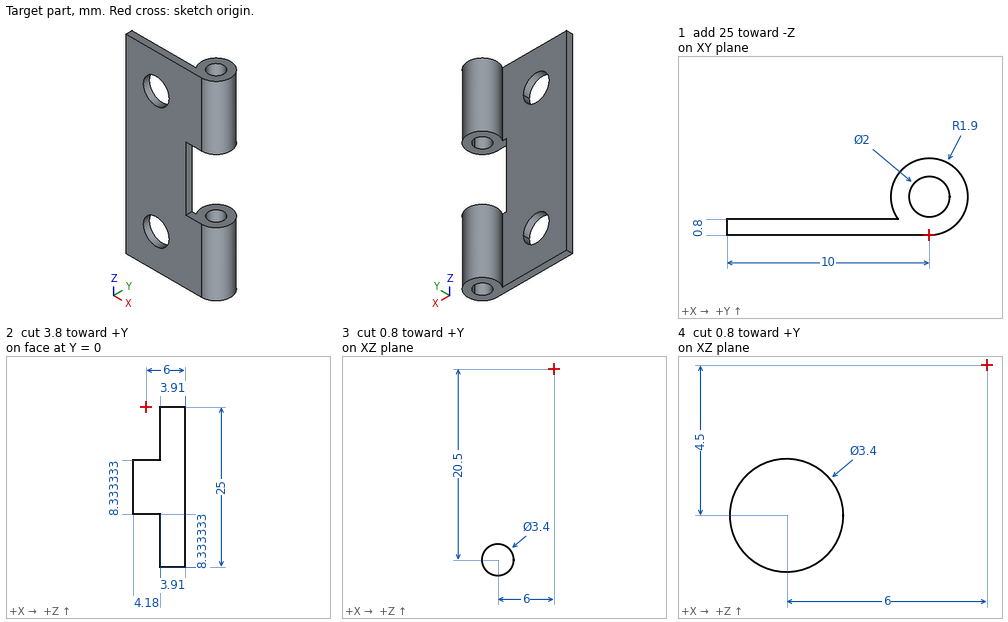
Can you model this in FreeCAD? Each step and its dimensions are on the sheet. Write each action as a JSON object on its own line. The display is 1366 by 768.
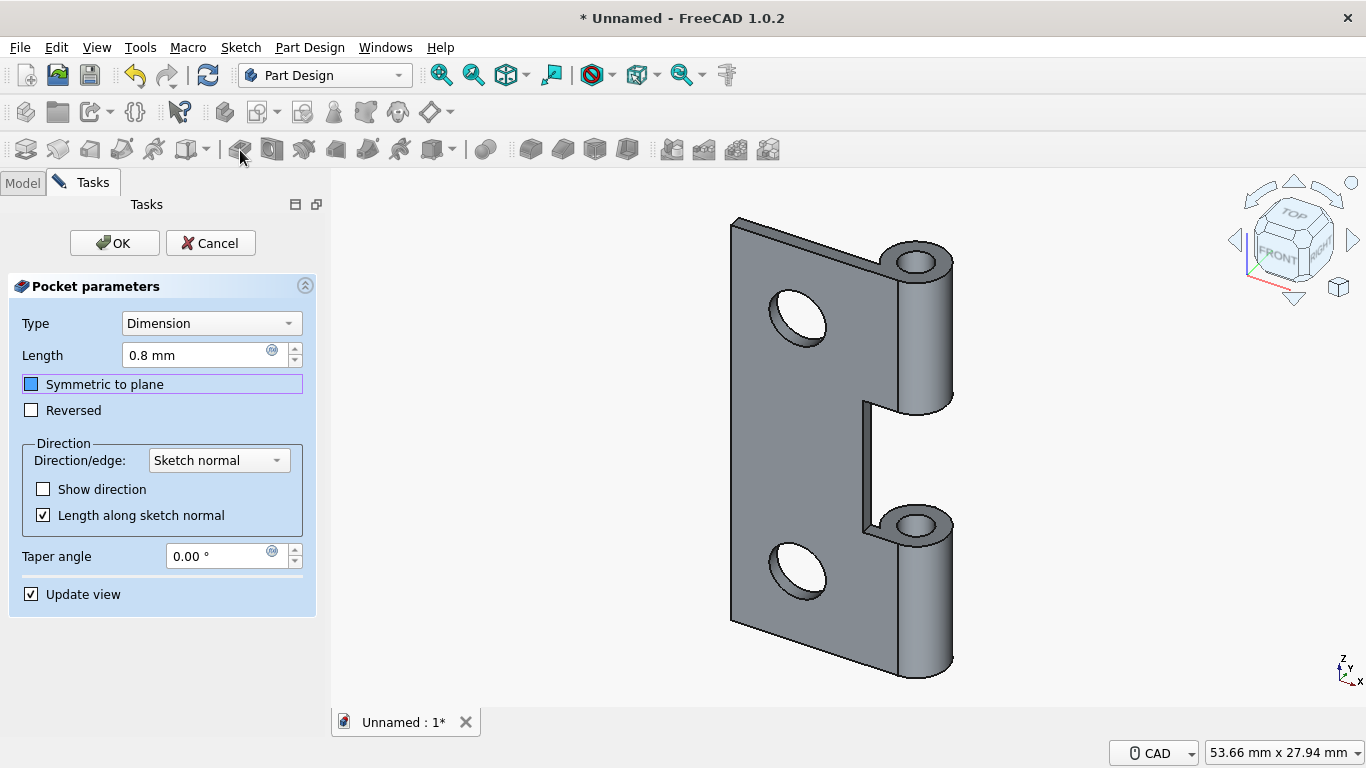
{"action": "left_click", "coordinate": [115, 243]}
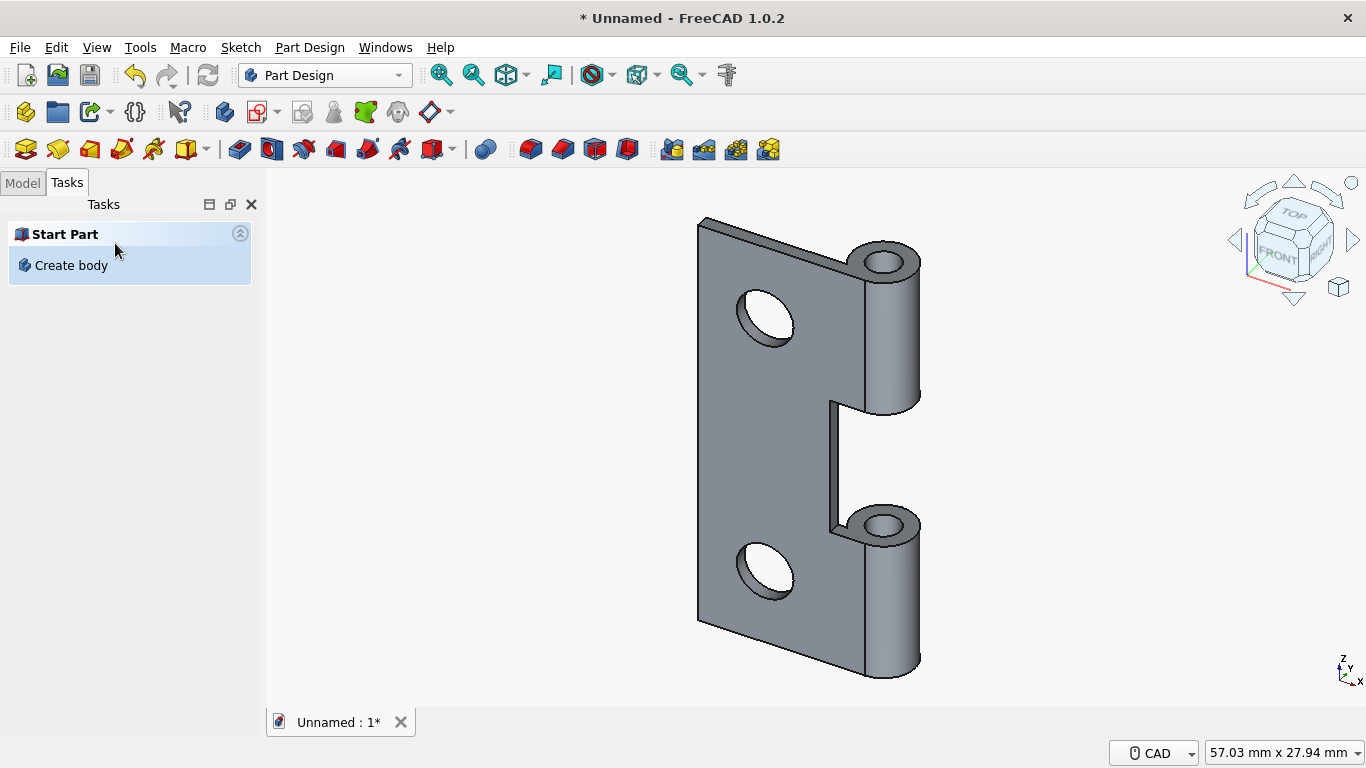
{"action": "key", "text": "0"}